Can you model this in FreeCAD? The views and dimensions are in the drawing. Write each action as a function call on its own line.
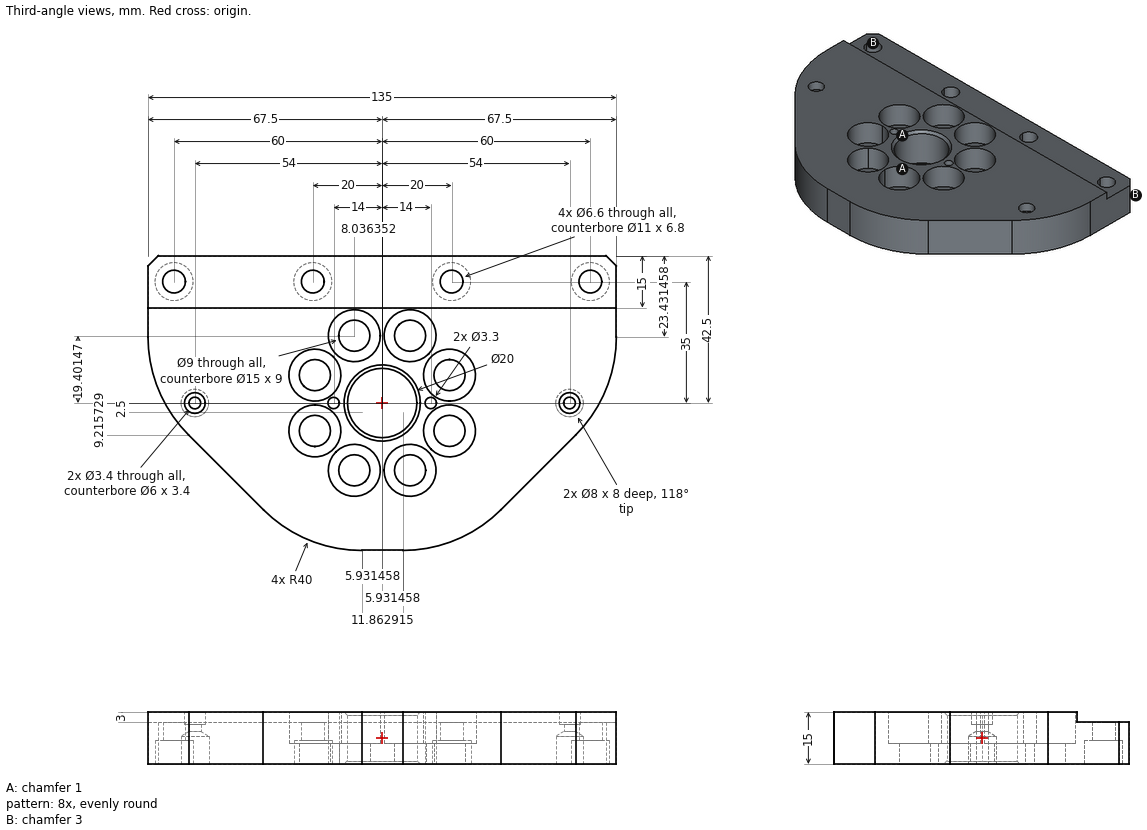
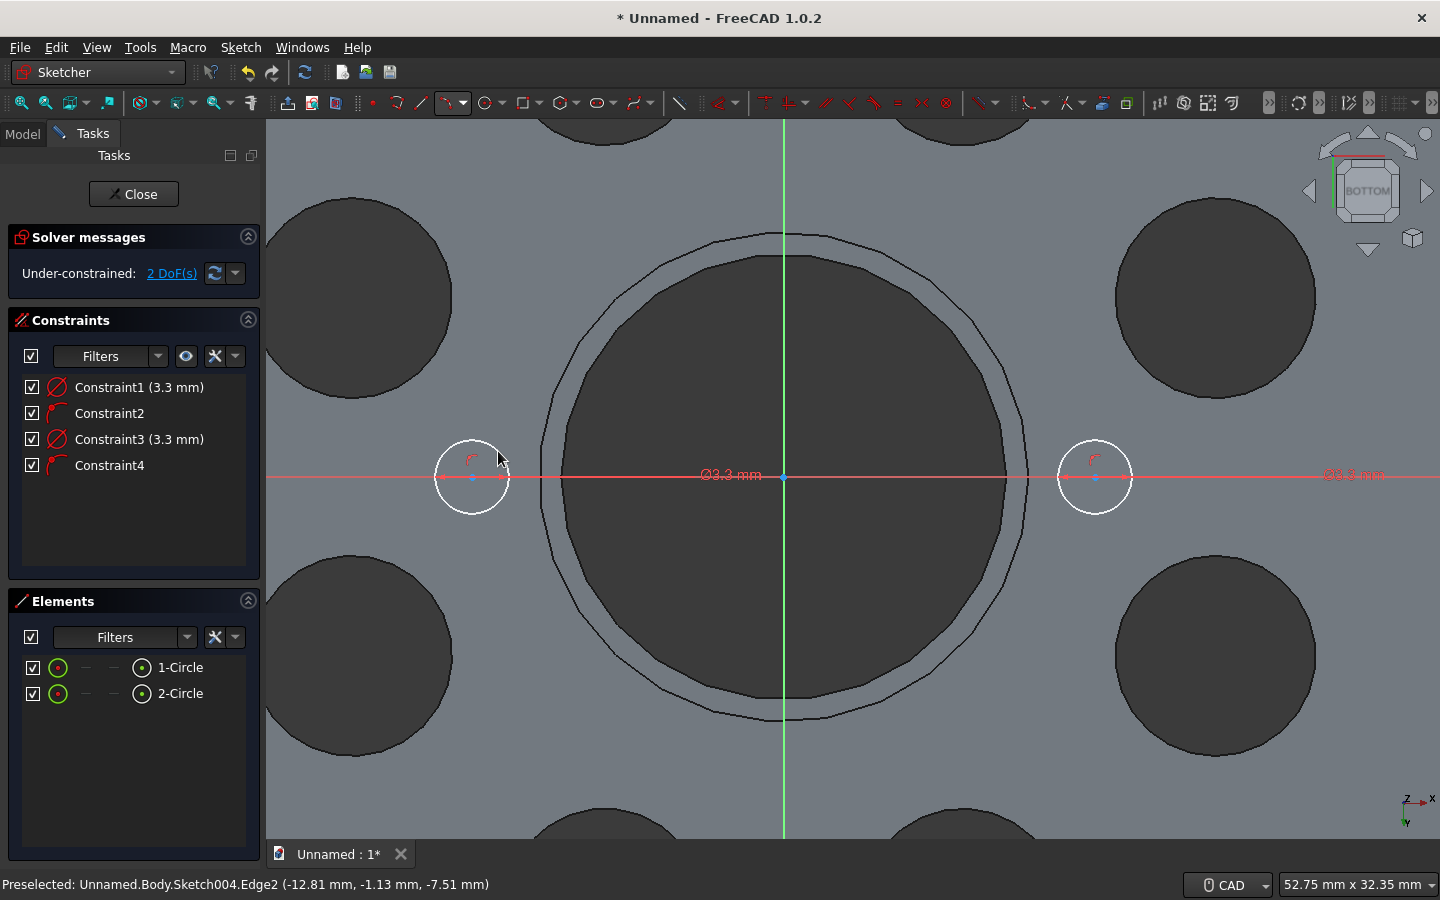
click(718, 104)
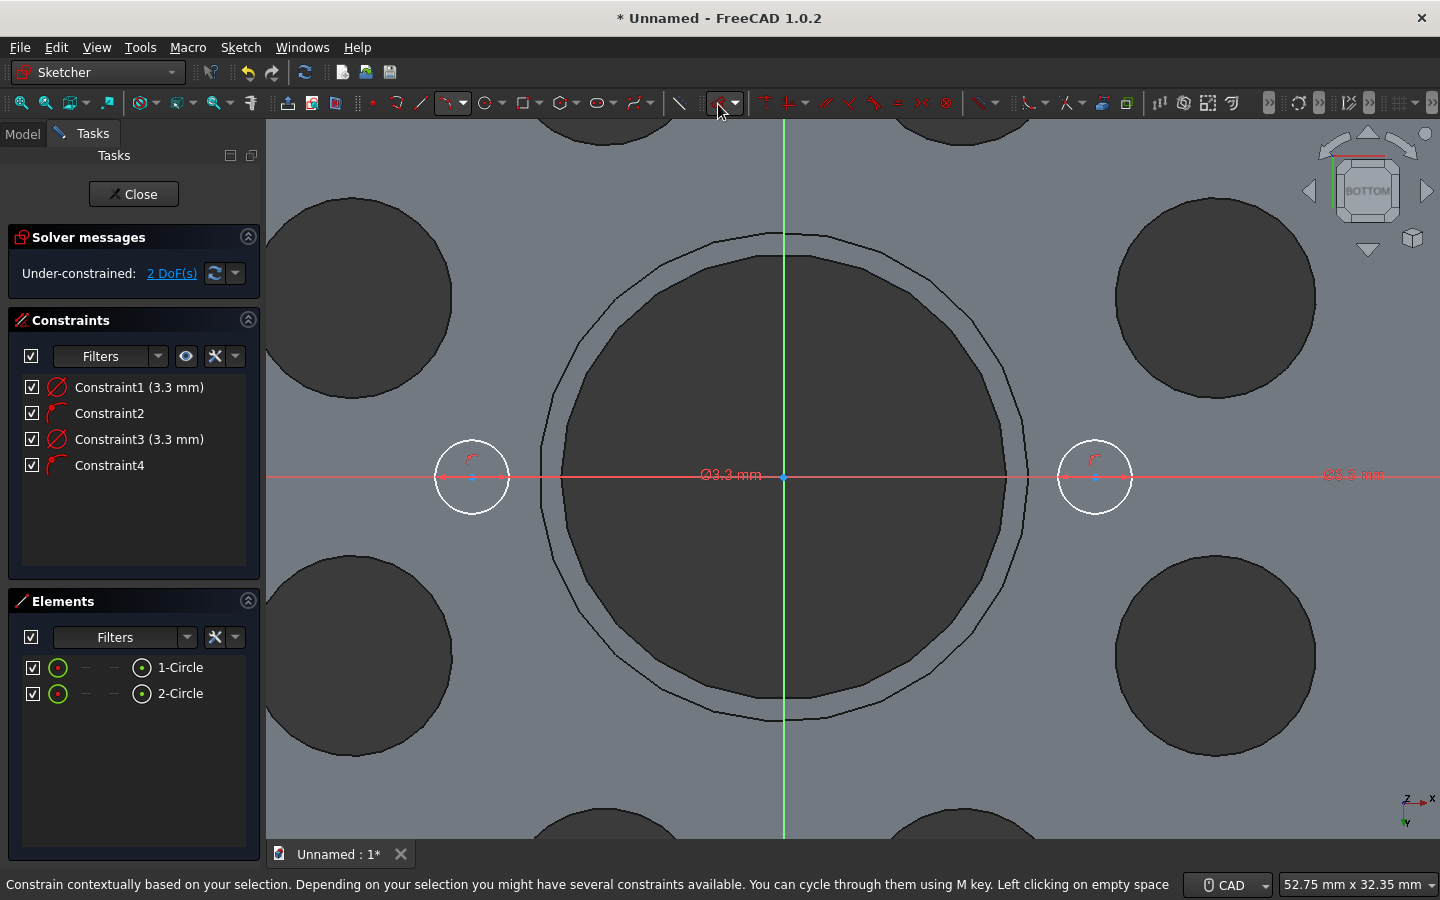
click(1095, 477)
click(939, 511)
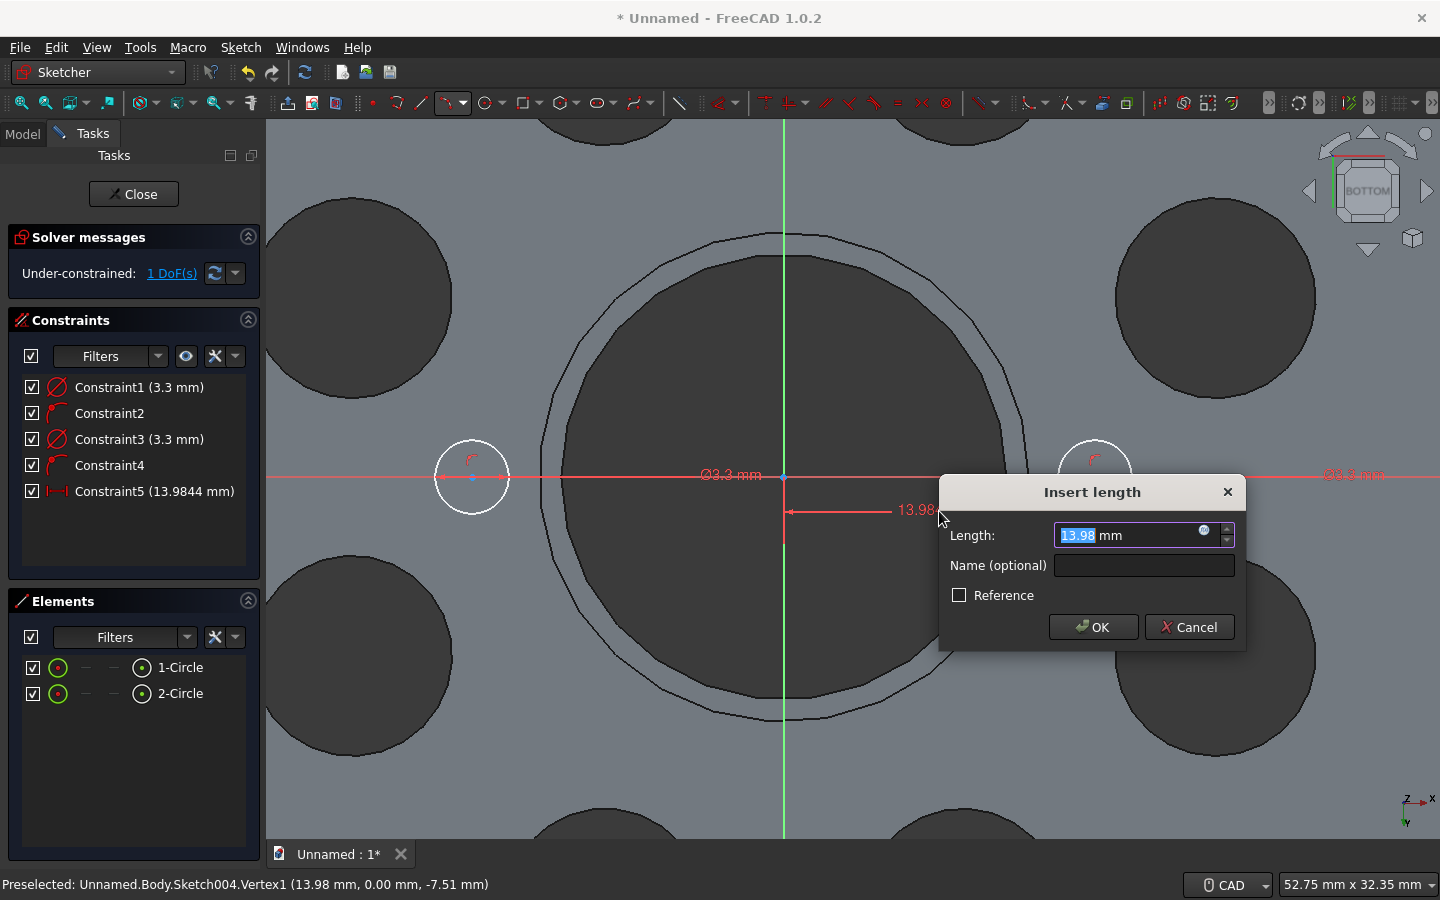
text(14)
key(Return)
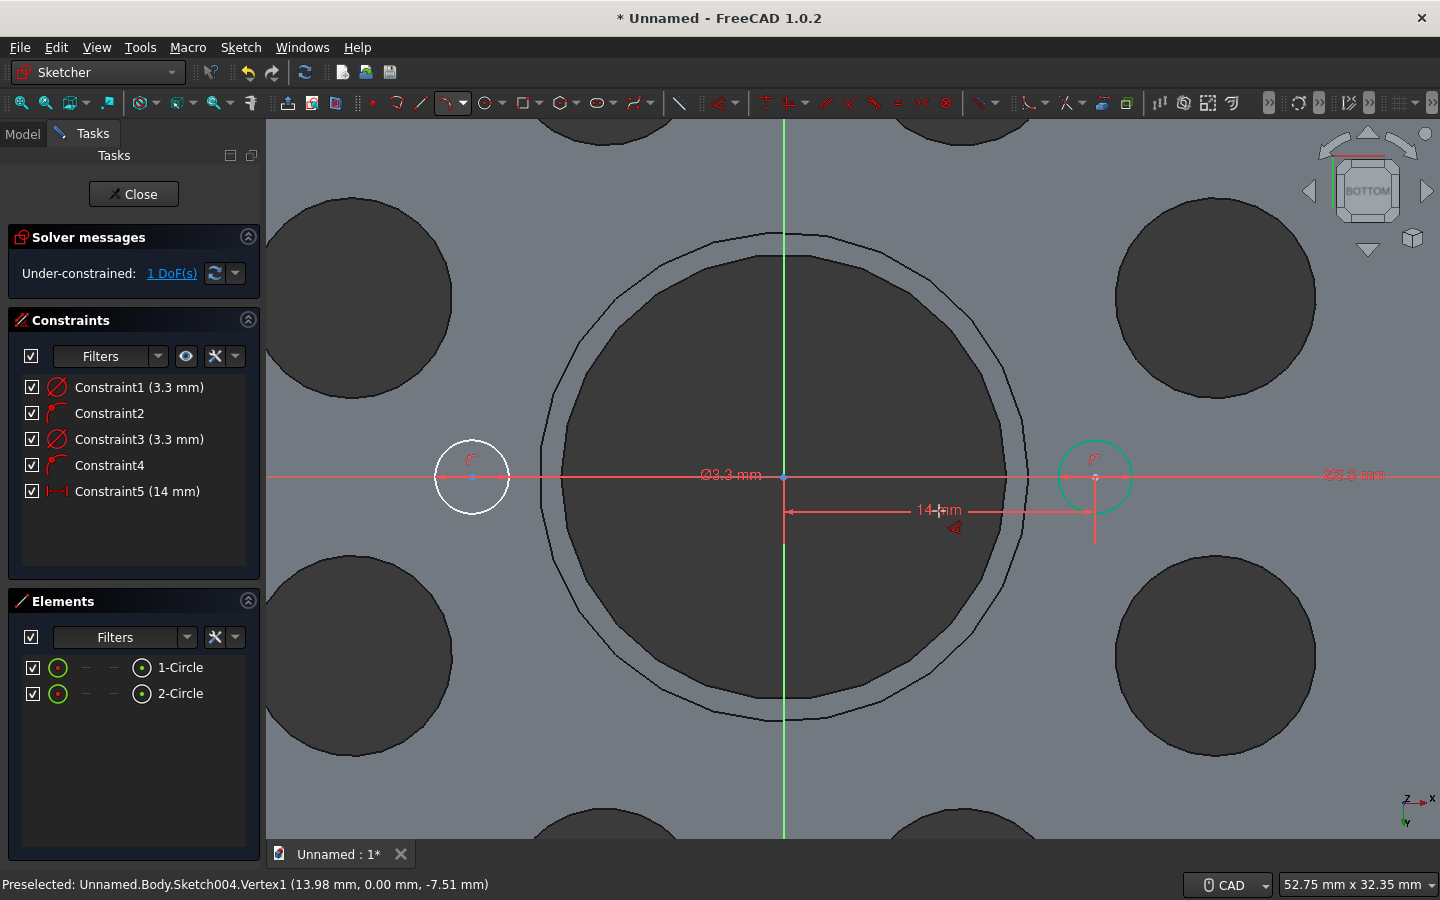
click(472, 477)
click(628, 511)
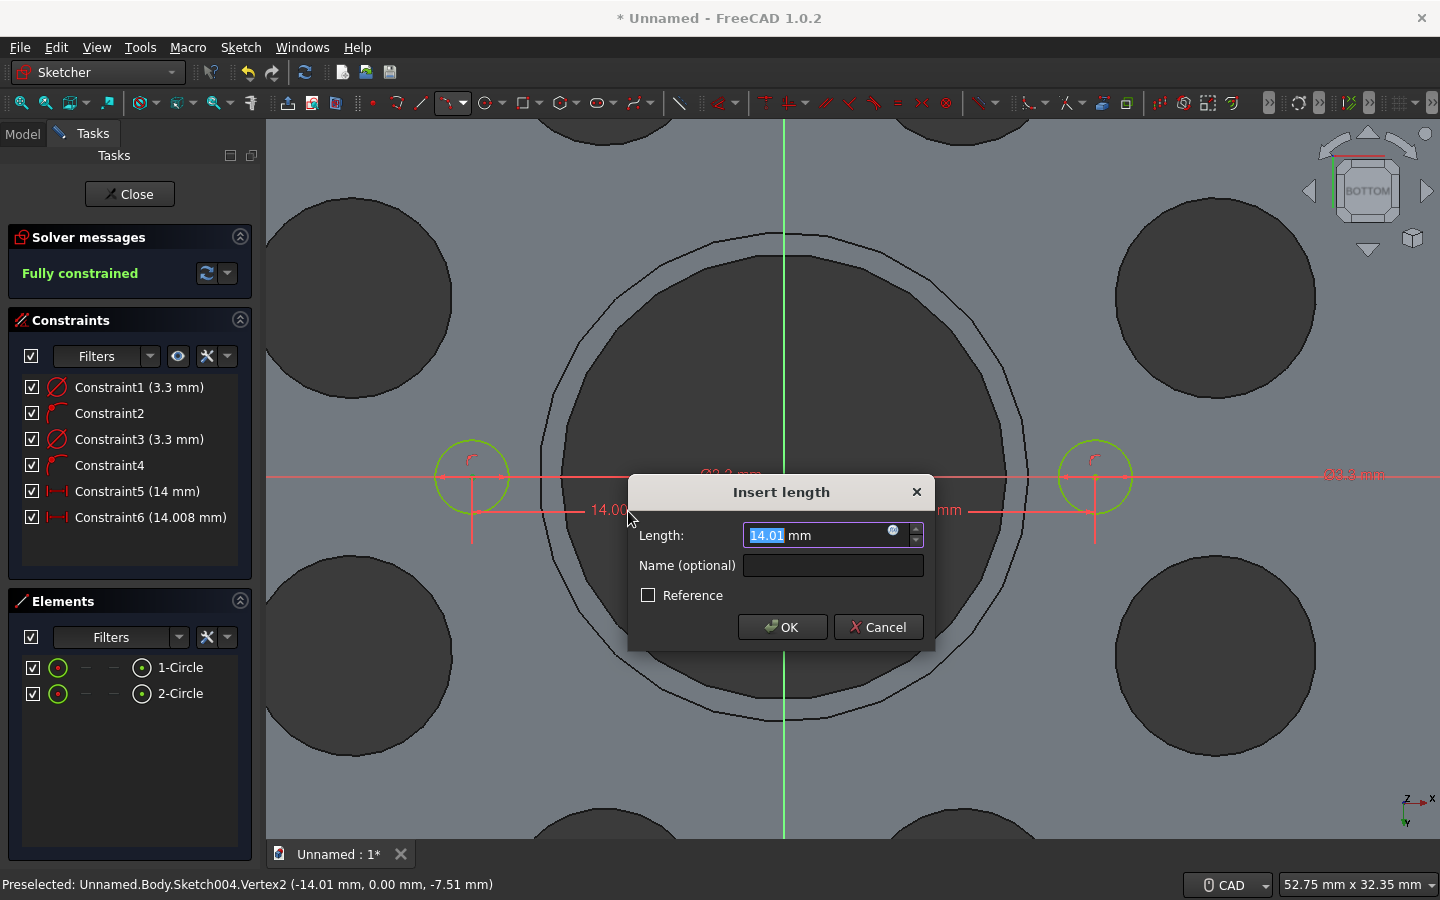
text(14)
key(Return)
key(Escape)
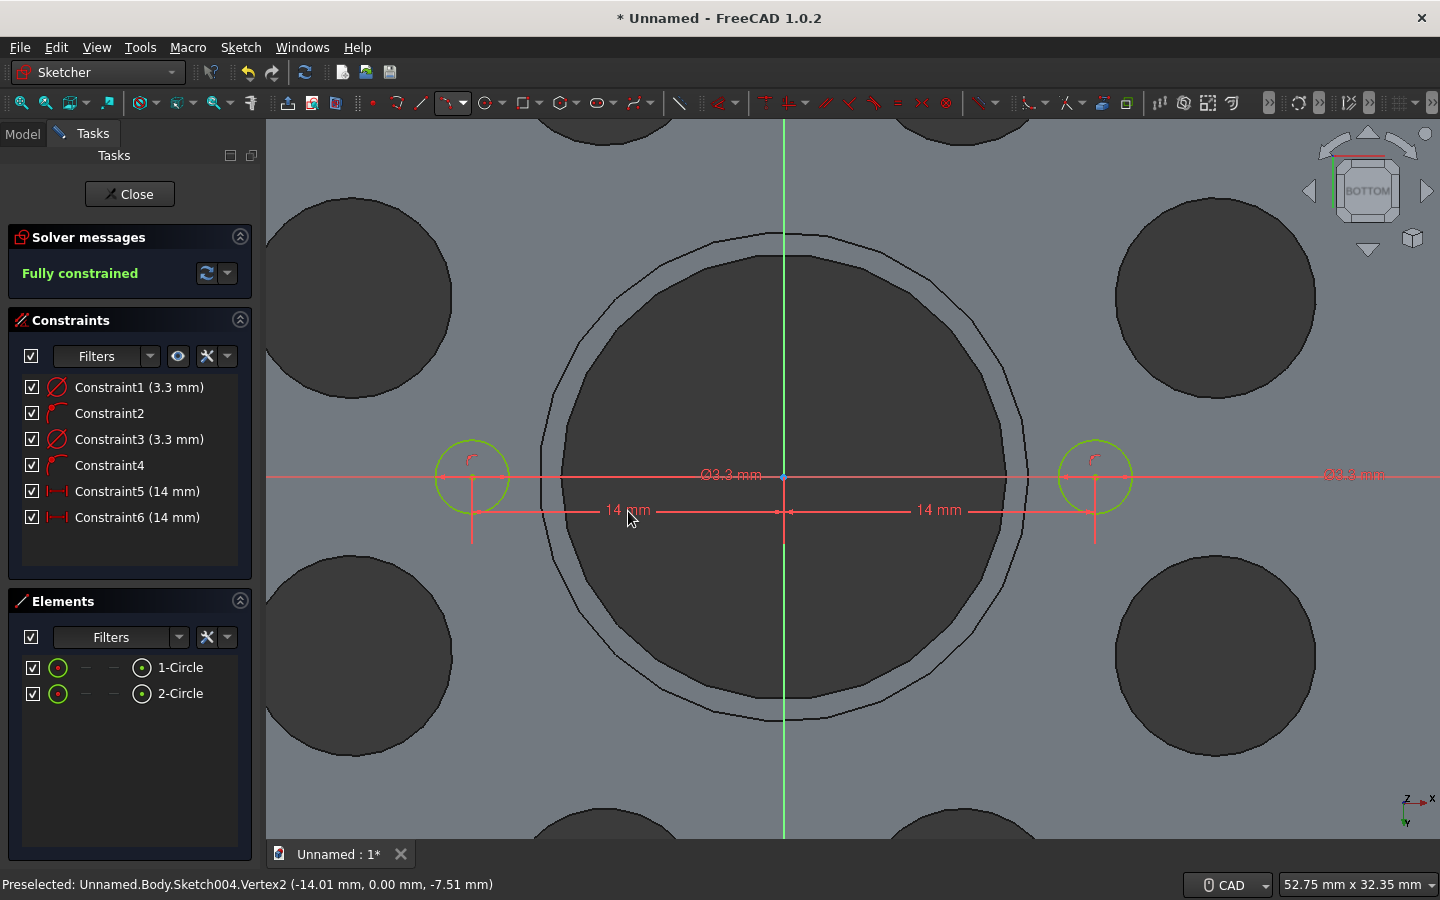
click(130, 194)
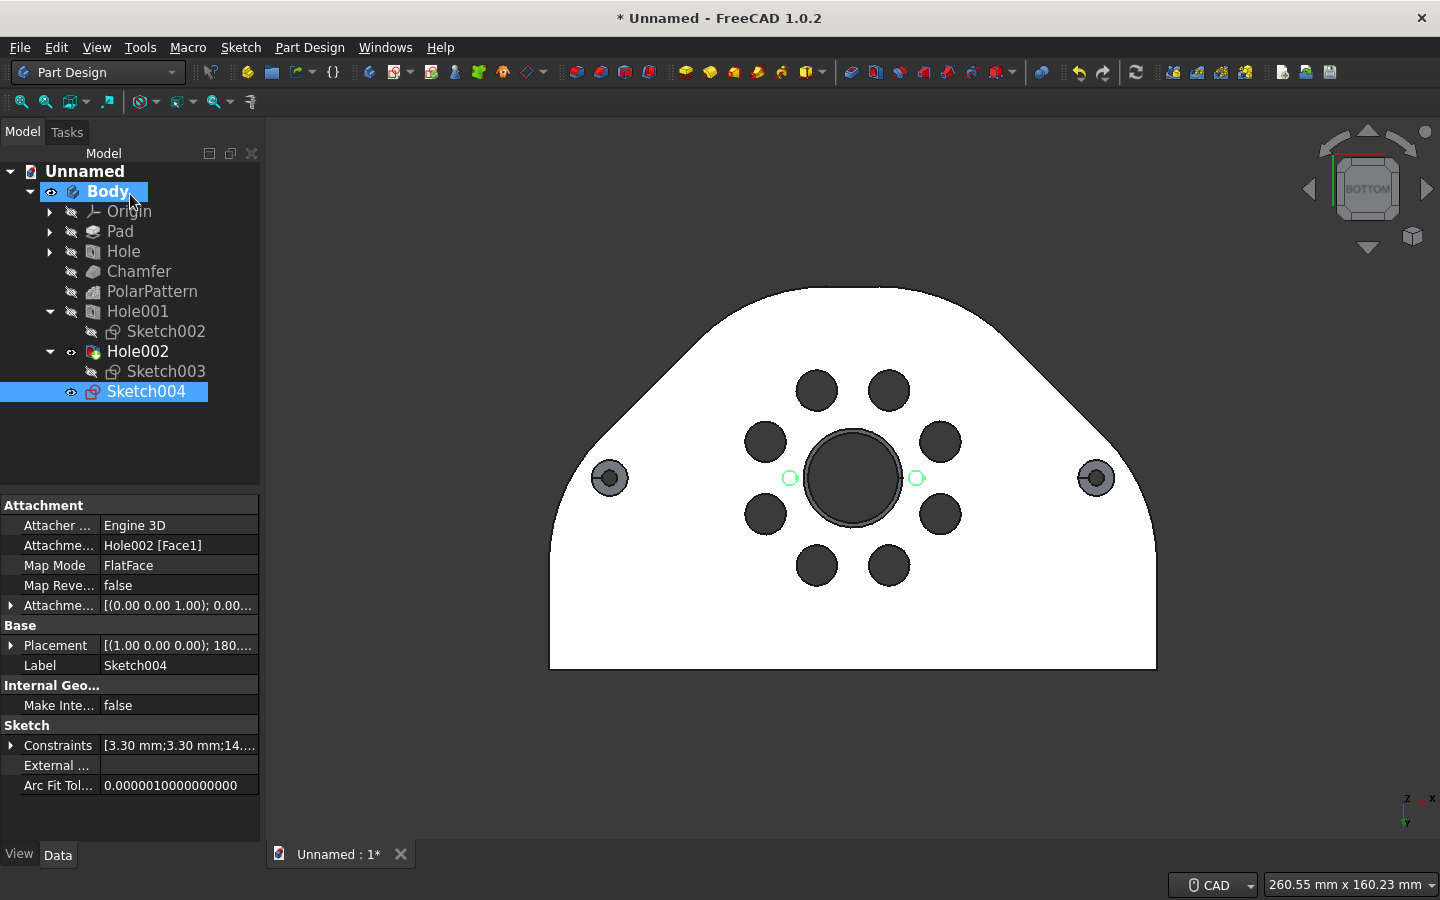
click(852, 72)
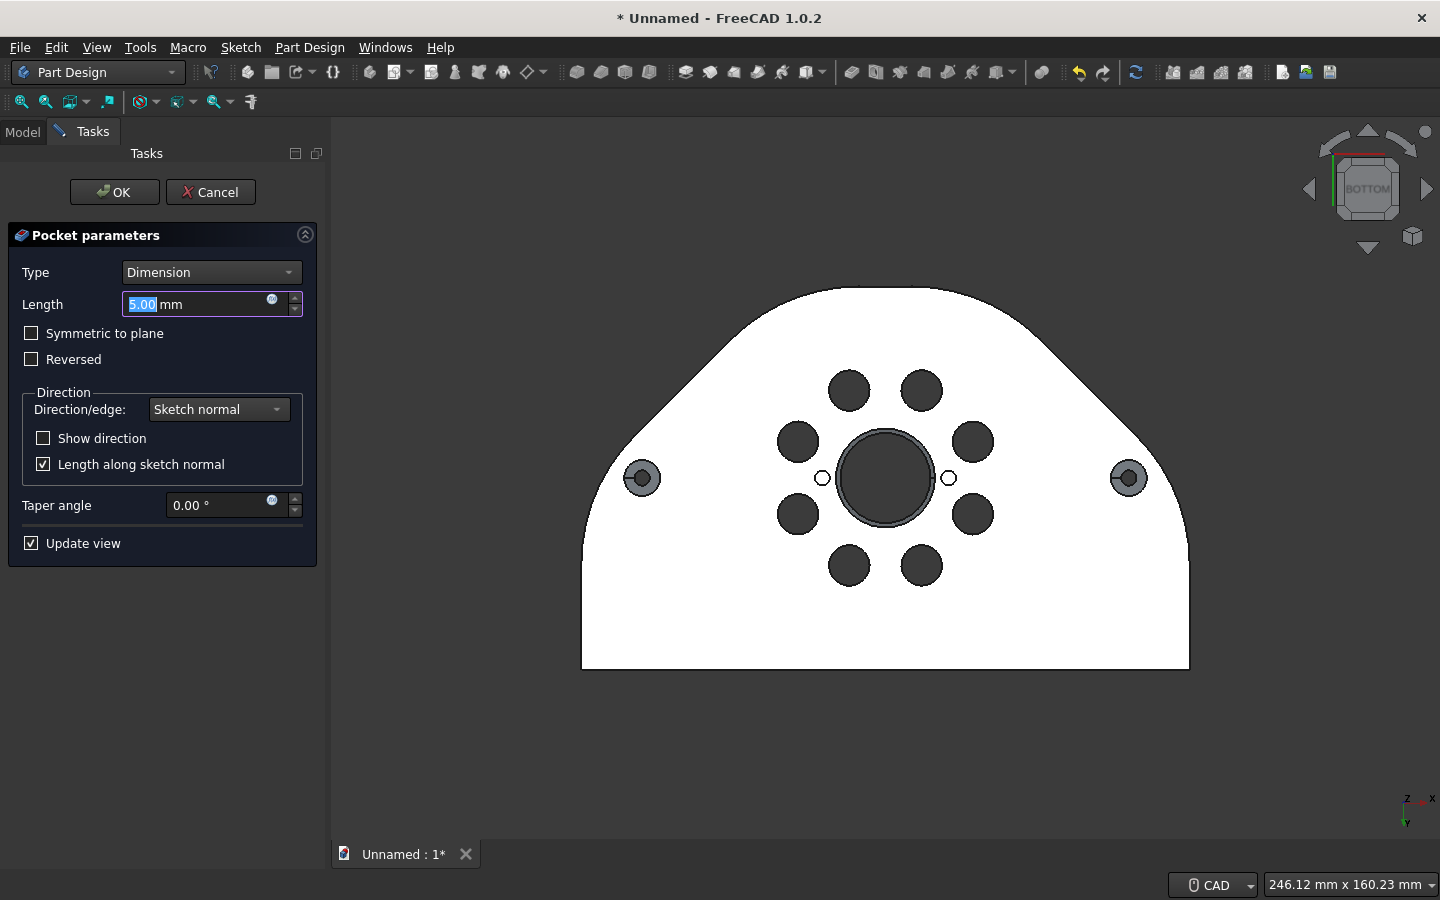
click(212, 272)